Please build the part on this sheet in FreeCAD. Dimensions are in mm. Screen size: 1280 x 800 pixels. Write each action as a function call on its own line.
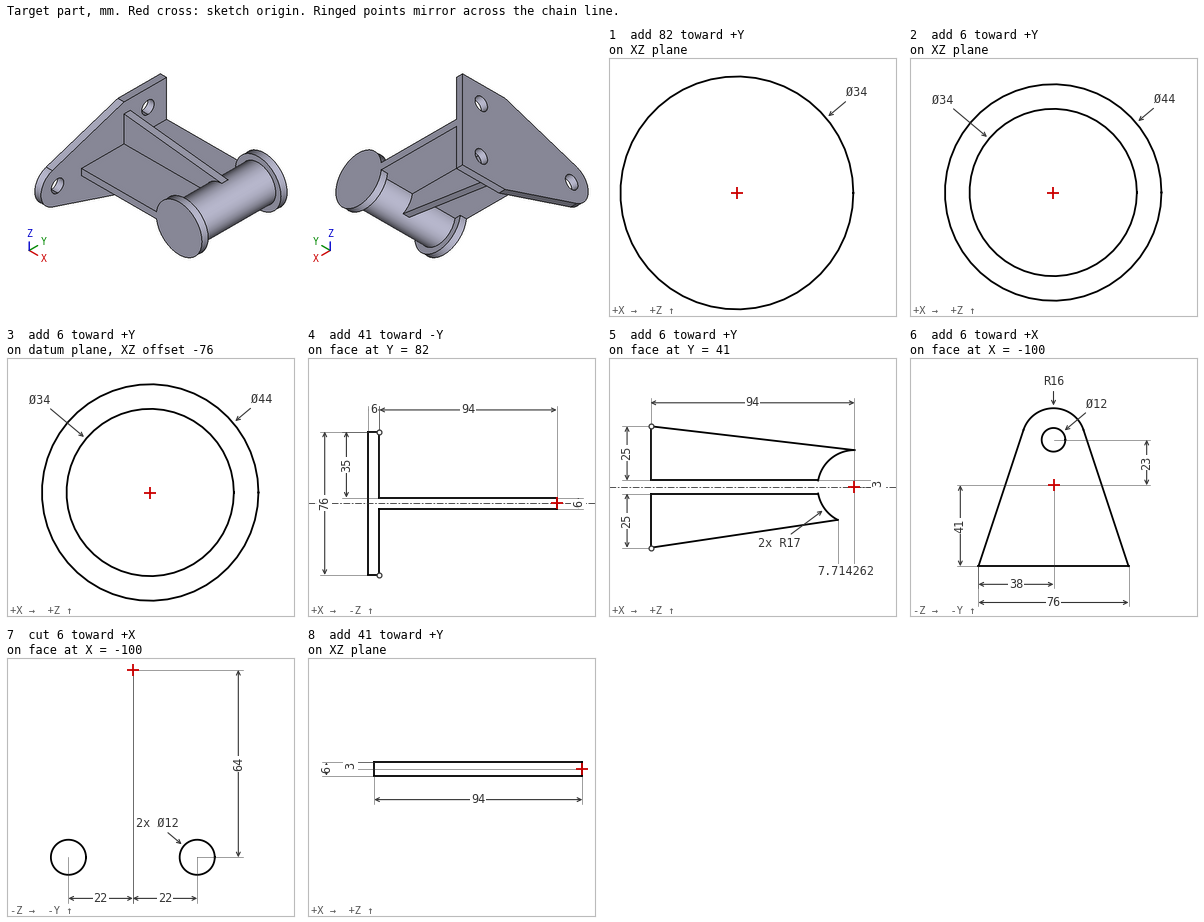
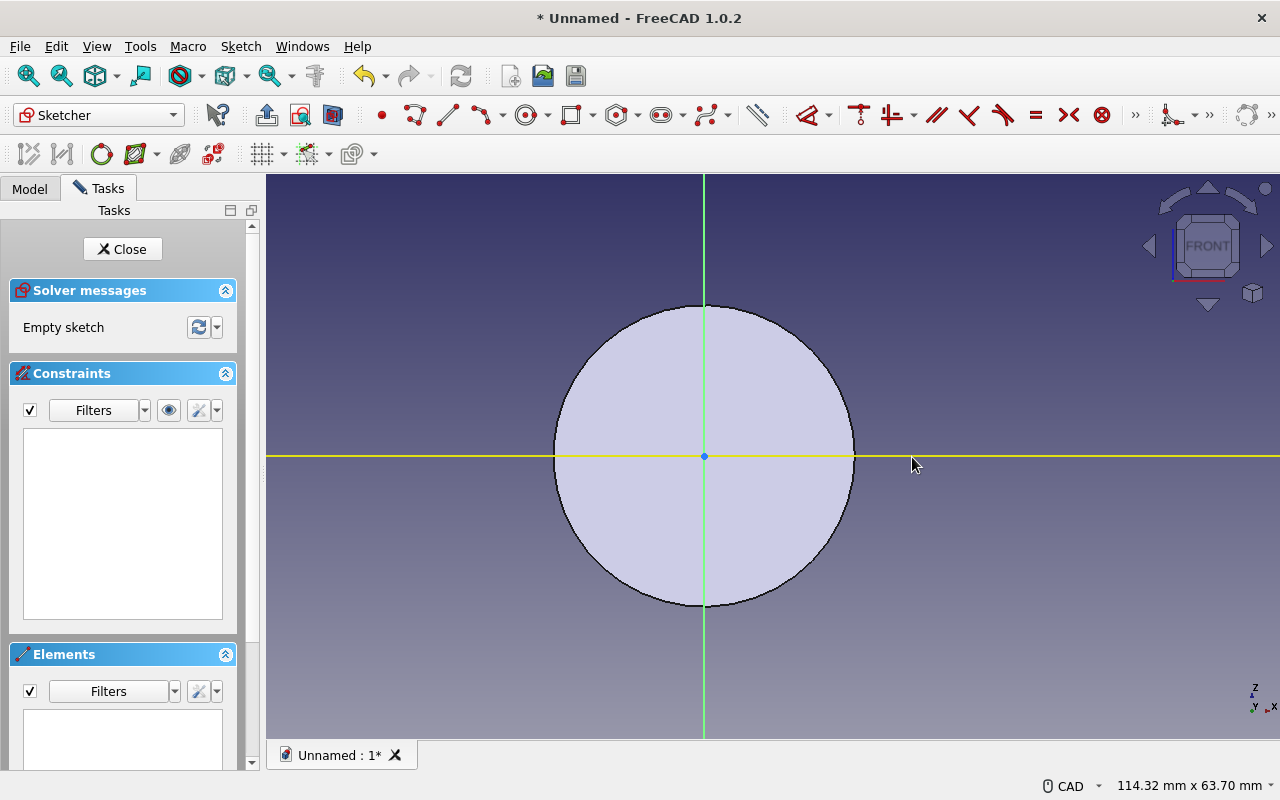
click(526, 116)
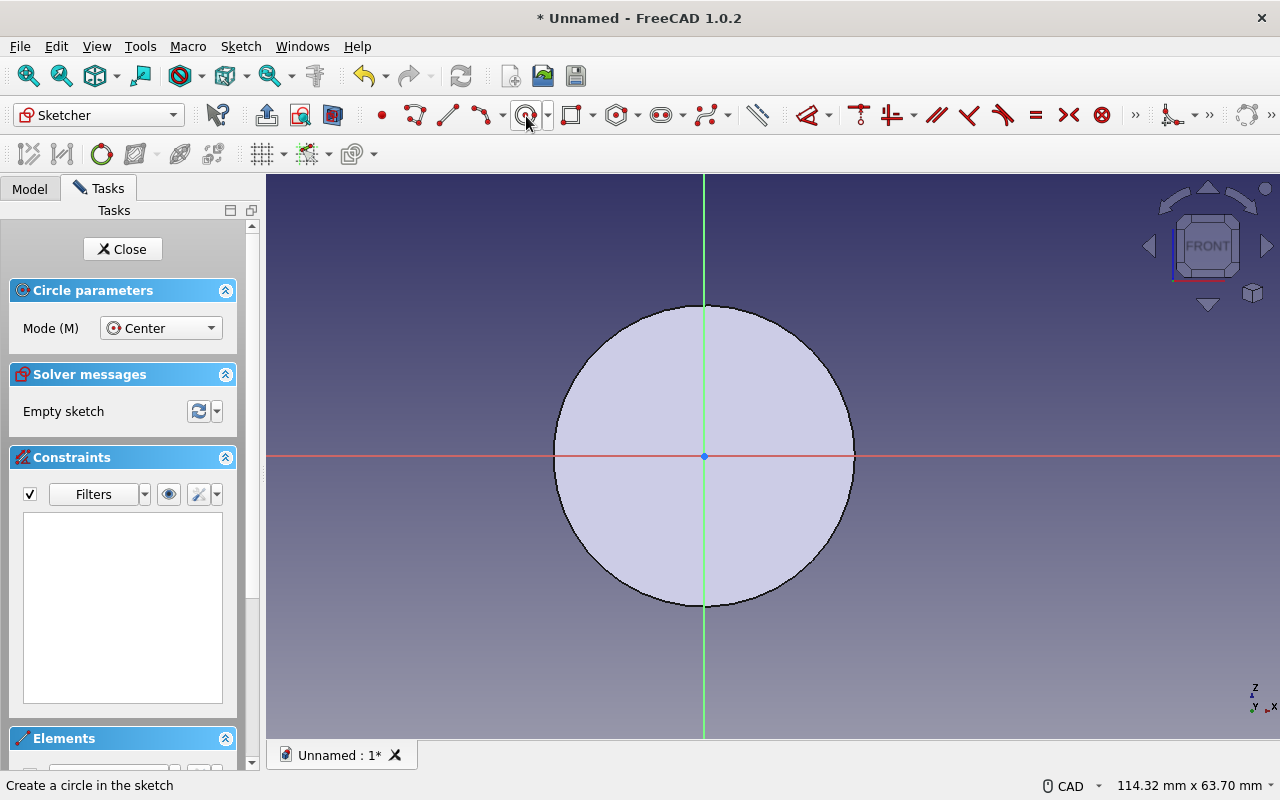
click(704, 456)
click(842, 318)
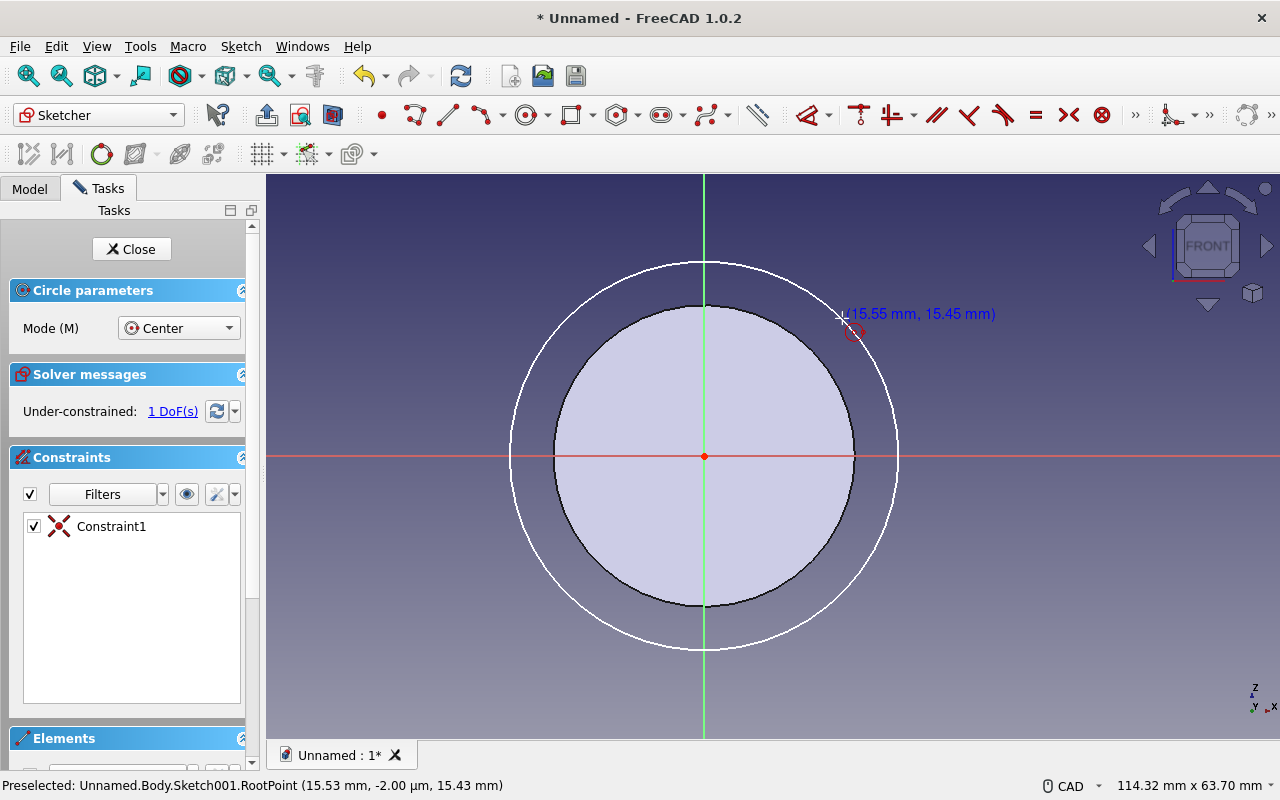
click(704, 456)
click(811, 349)
key(Escape)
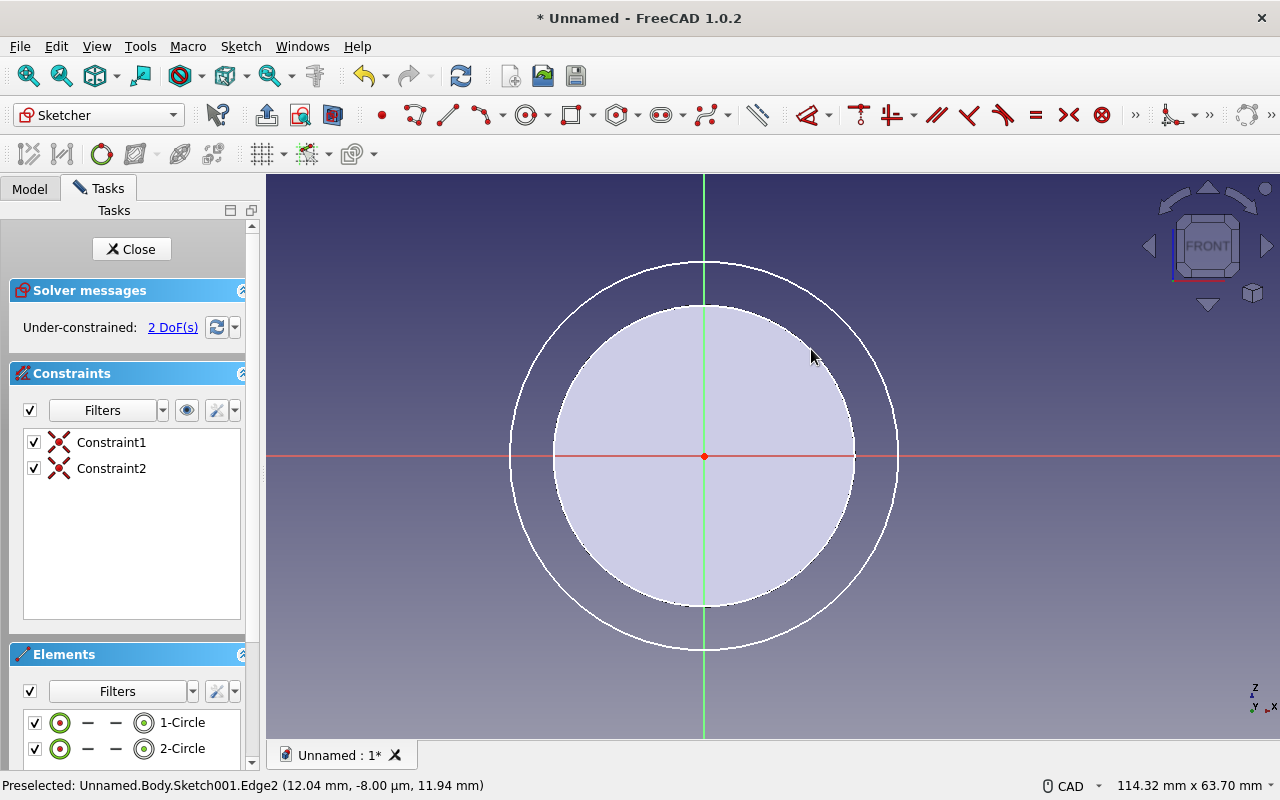
click(806, 116)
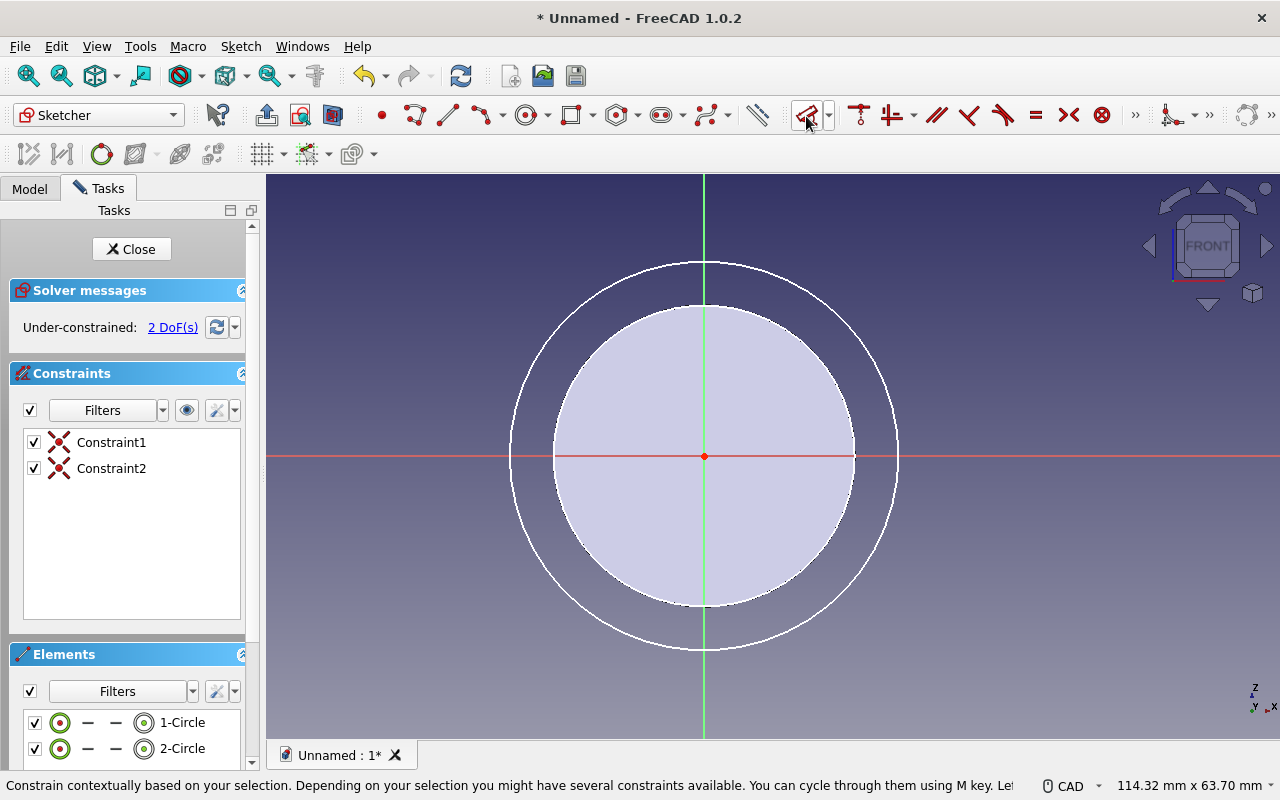
click(841, 318)
click(864, 295)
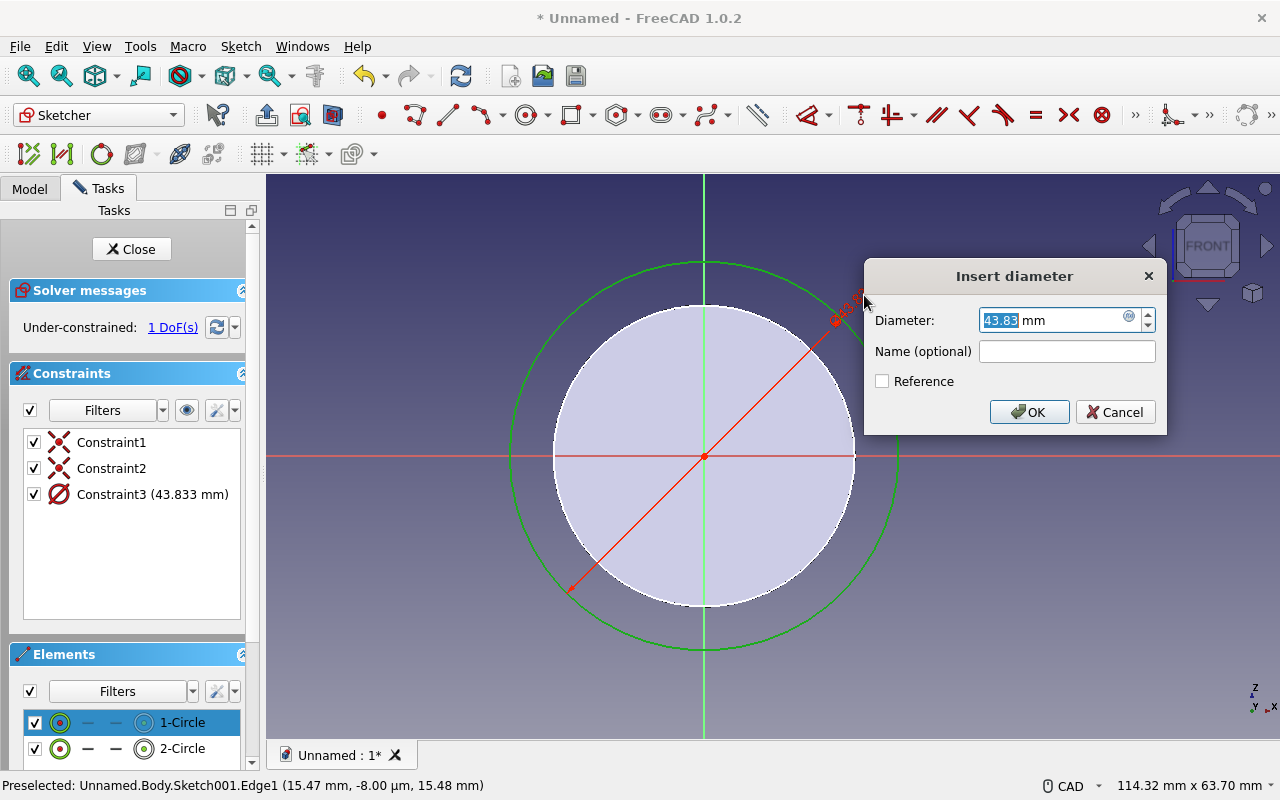
text(44)
key(Return)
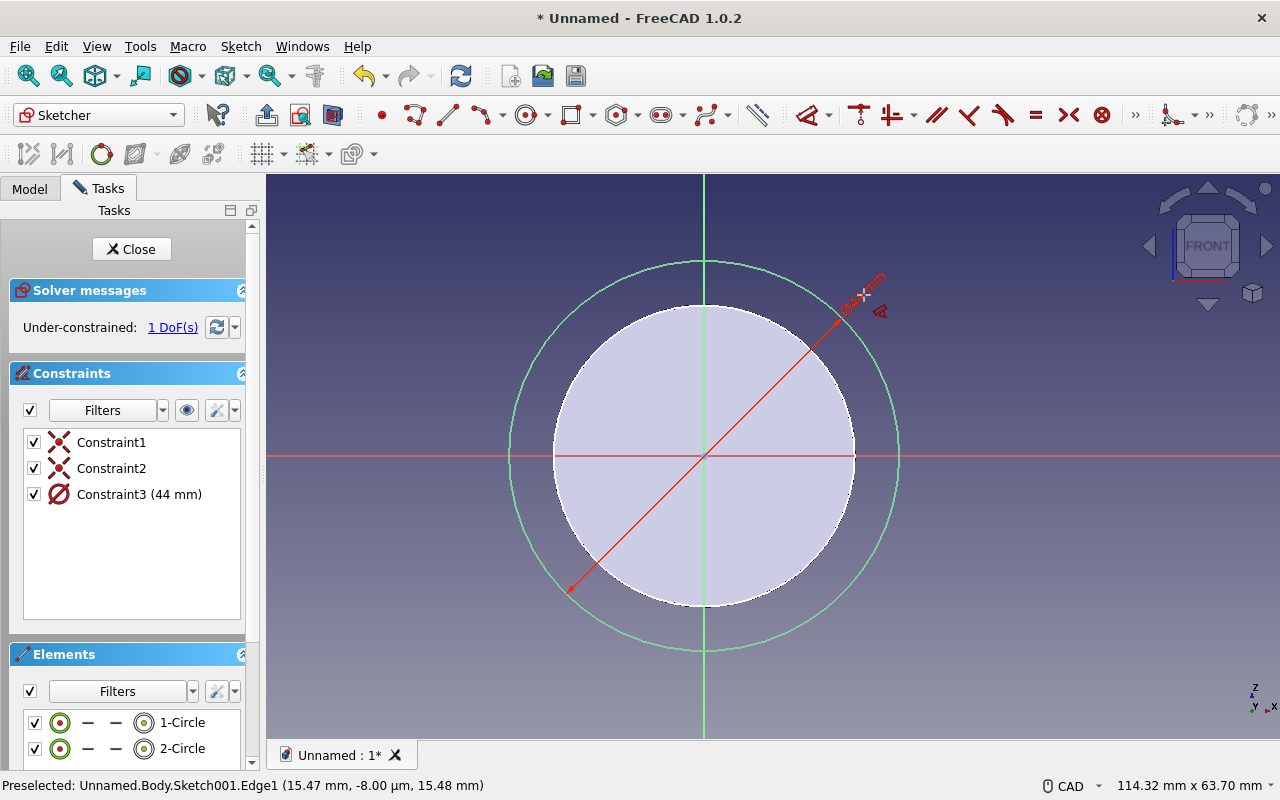
click(810, 349)
click(925, 390)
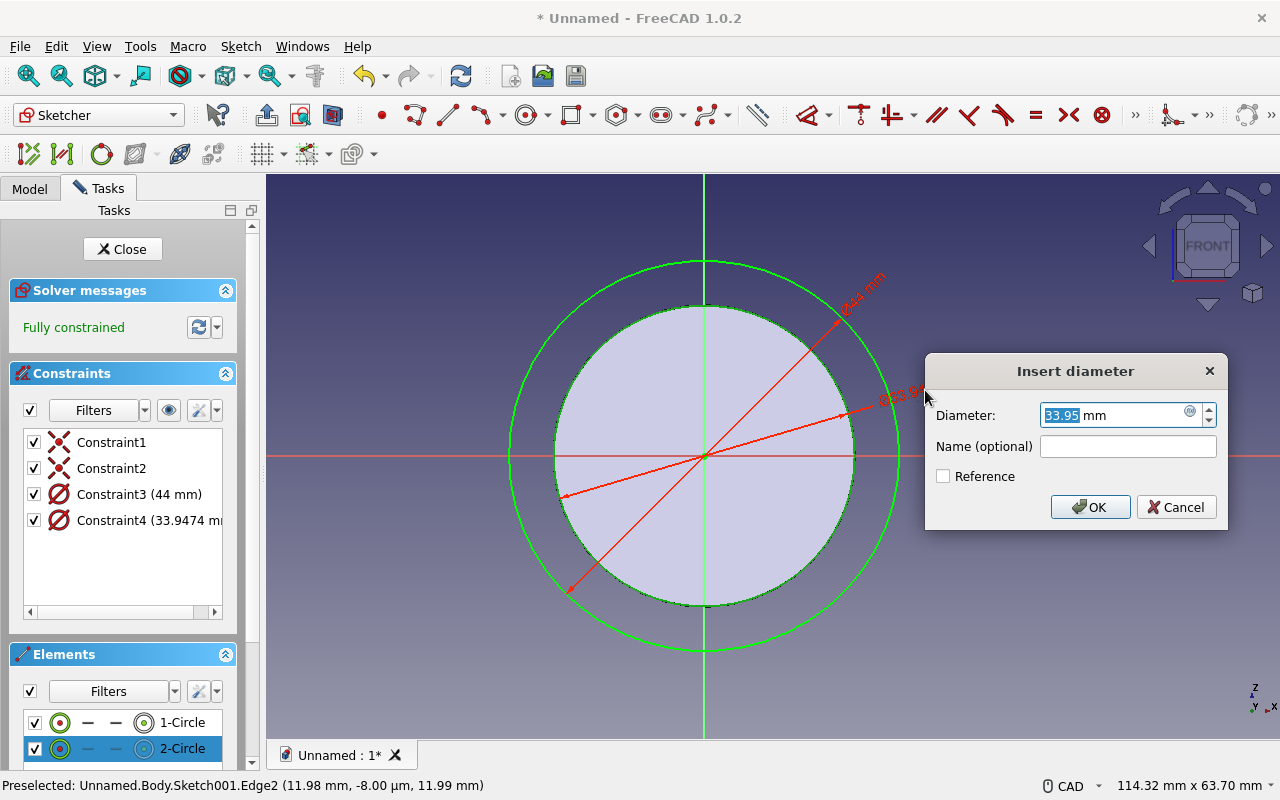
text(34)
key(Return)
key(Escape)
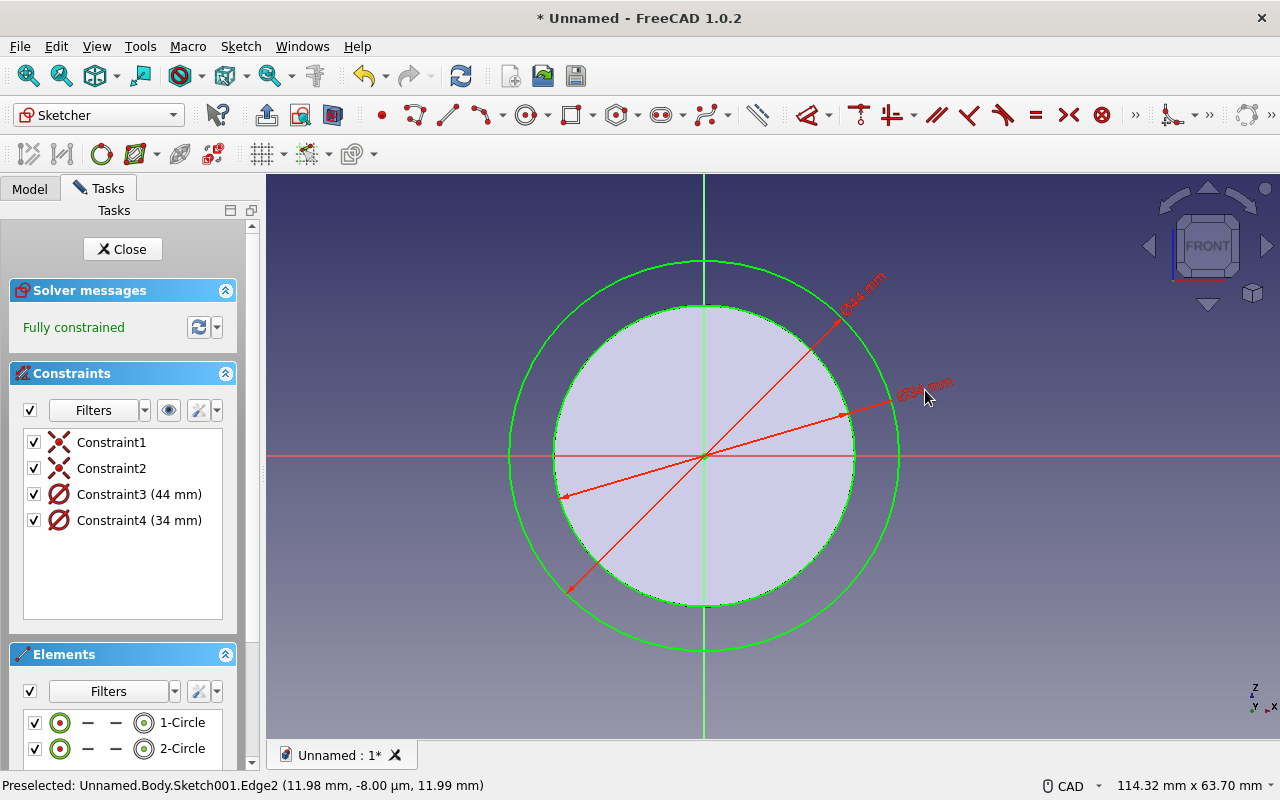
click(123, 249)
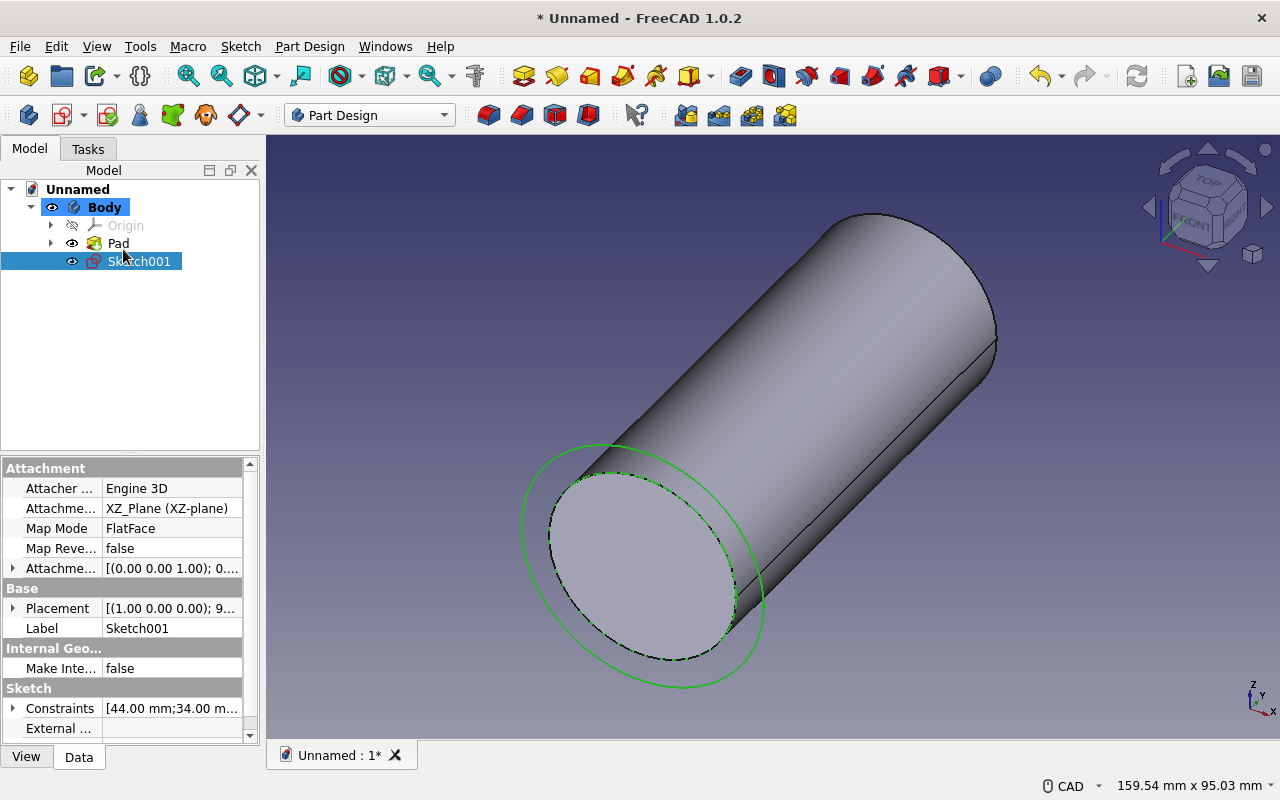
click(524, 76)